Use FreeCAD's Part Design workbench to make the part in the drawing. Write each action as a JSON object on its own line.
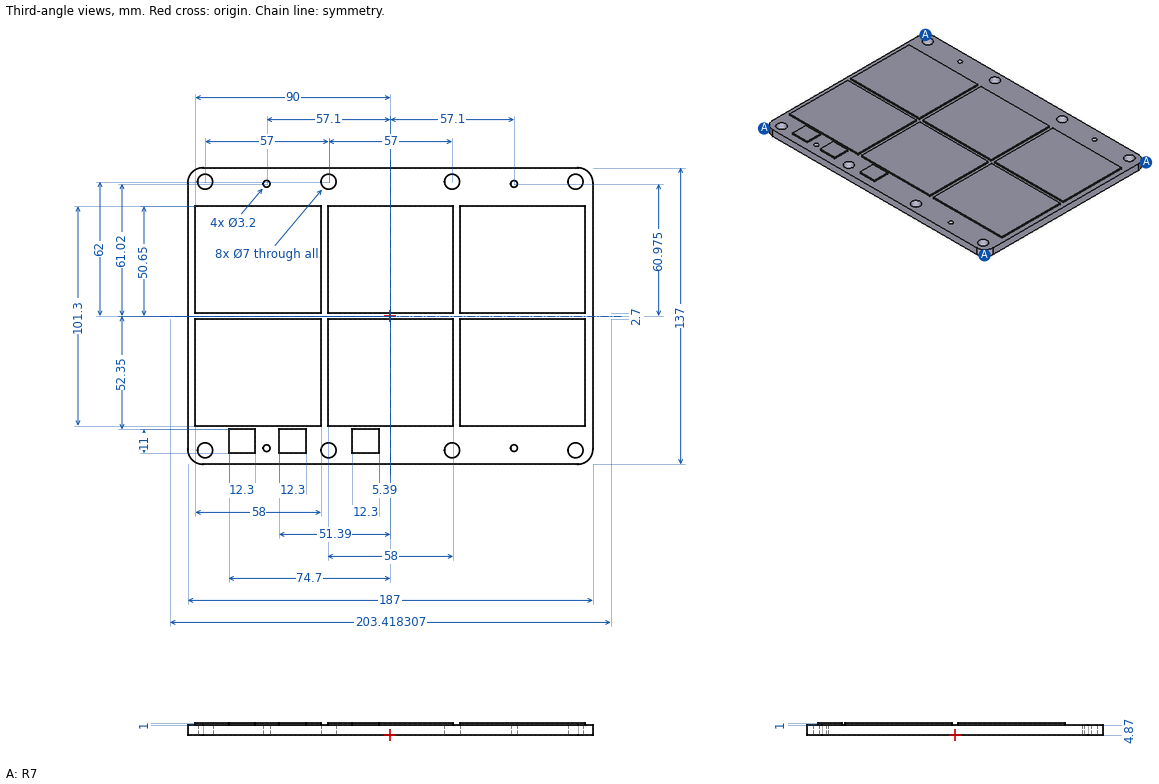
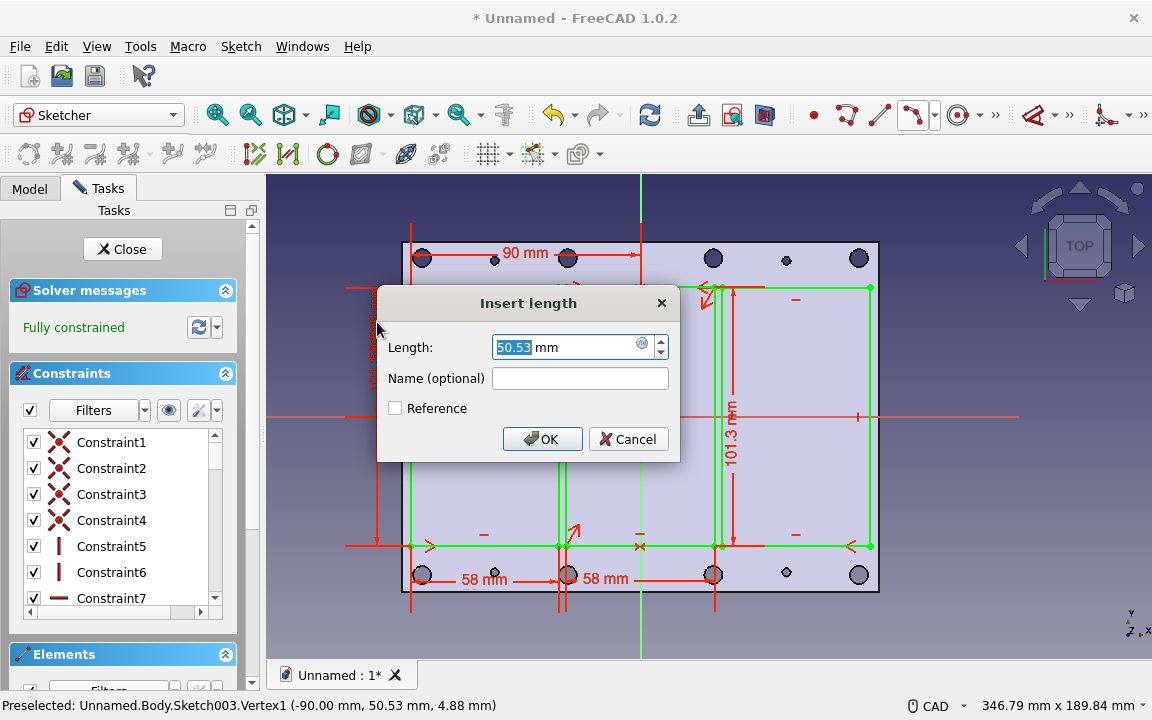
{"action": "type", "text": "50.65"}
{"action": "key", "text": "Return"}
{"action": "key", "text": "Escape"}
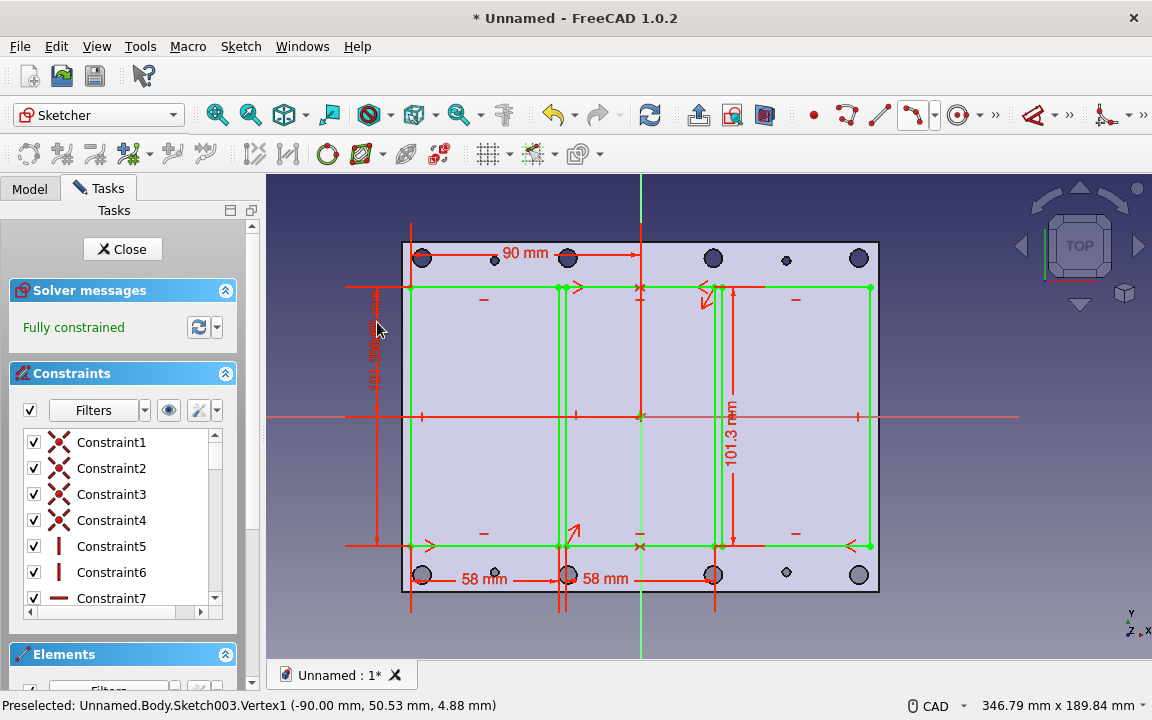
{"action": "left_click", "coordinate": [123, 249]}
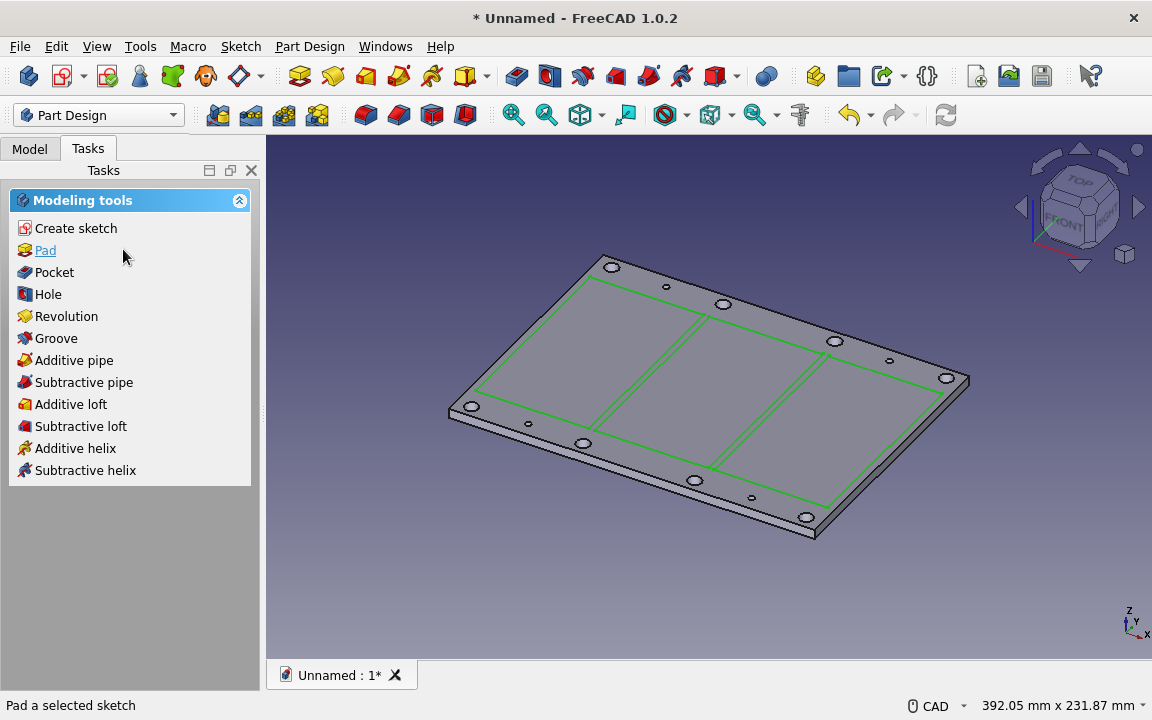
{"action": "left_click", "coordinate": [300, 76]}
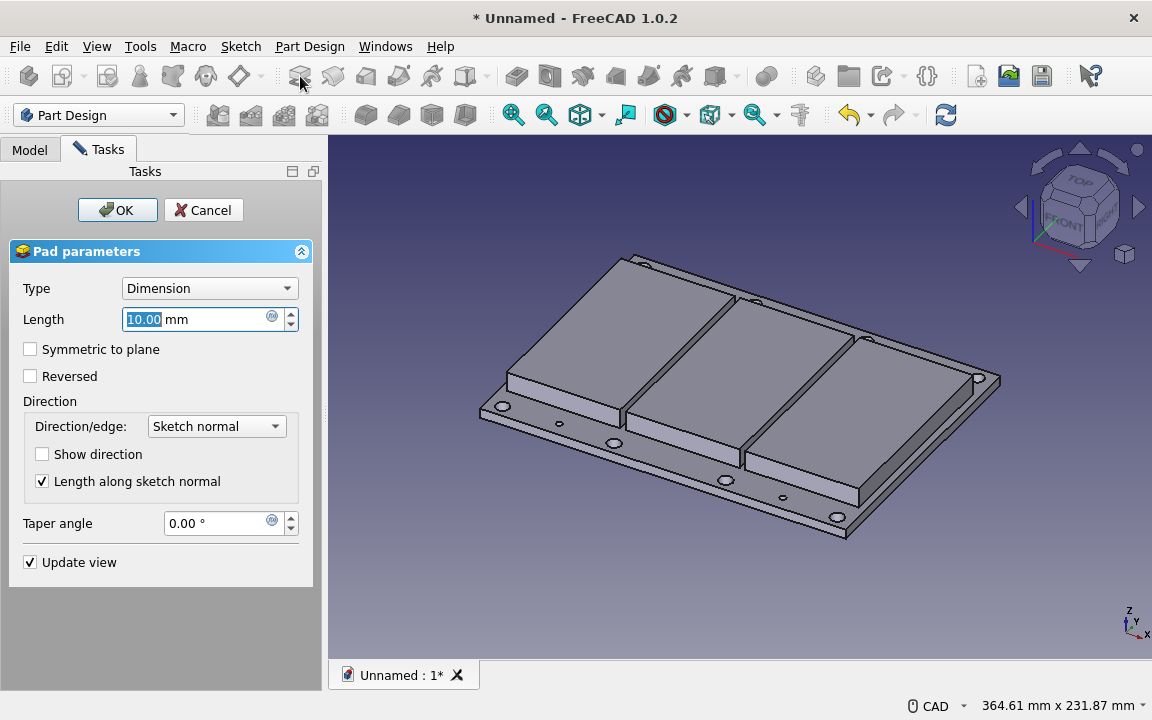
{"action": "type", "text": "1"}
{"action": "key", "text": "Tab"}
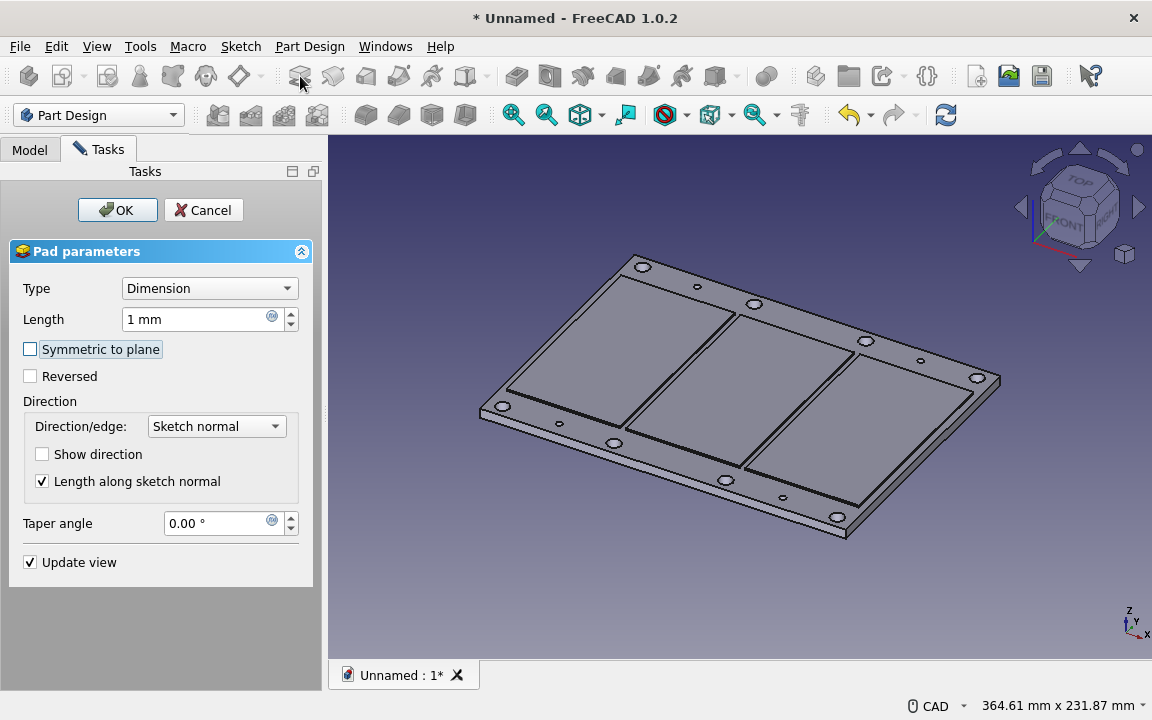
{"action": "left_click", "coordinate": [118, 210]}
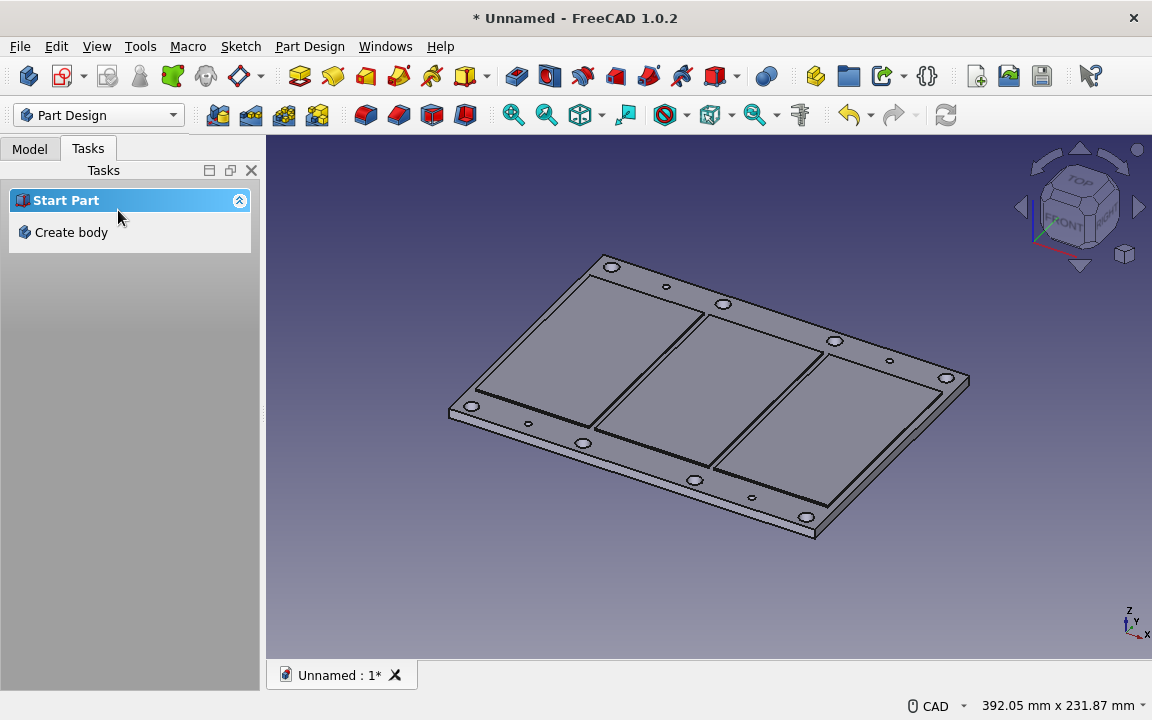
{"action": "left_click", "coordinate": [643, 457]}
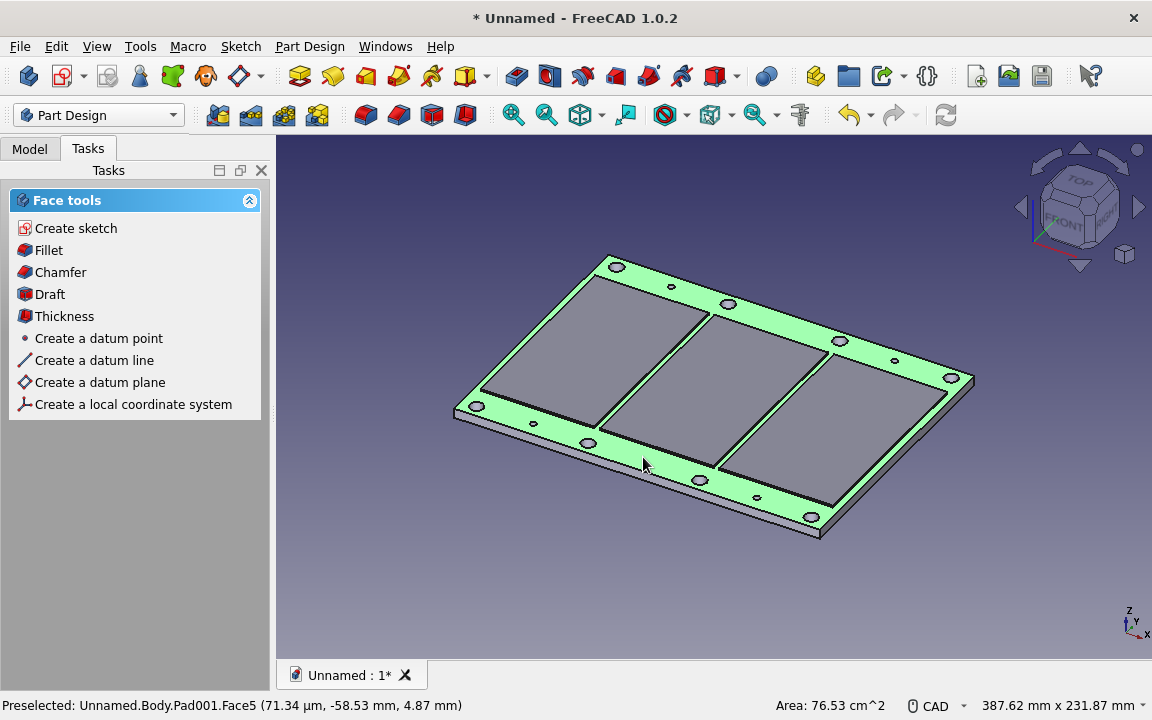
{"action": "left_click", "coordinate": [62, 76]}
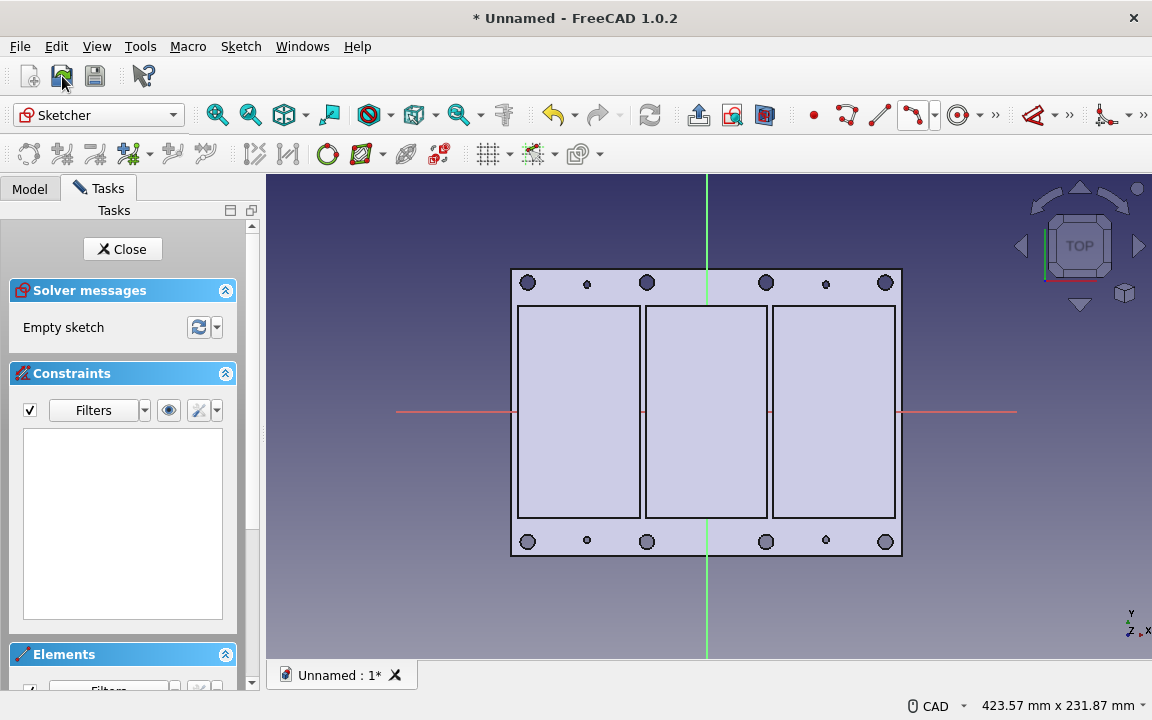
{"action": "key", "text": "q s"}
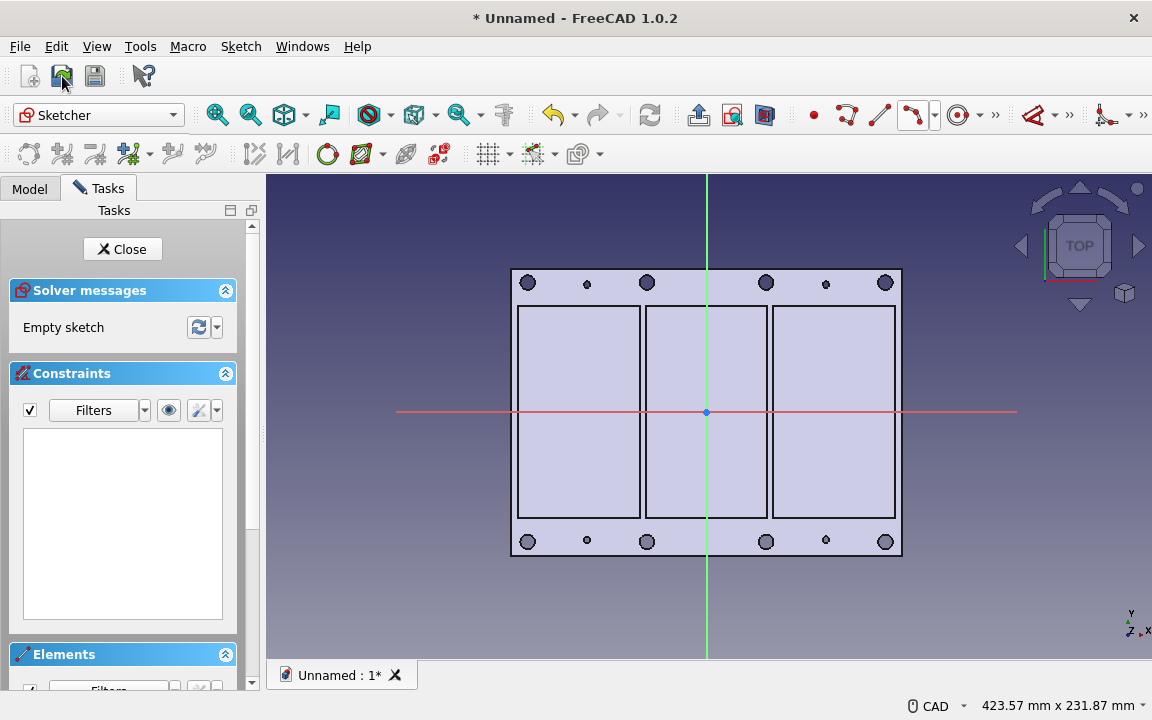
{"action": "scroll", "coordinate": [619, 529], "scroll_direction": "up", "scroll_amount": 4}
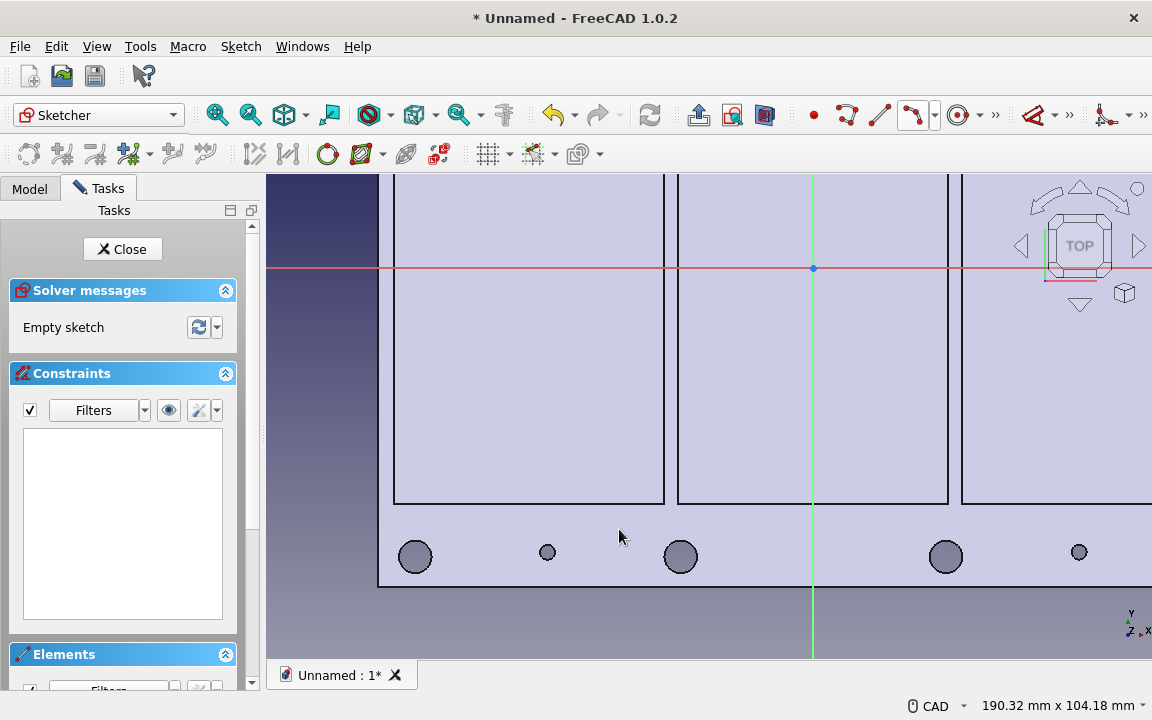
{"action": "key", "text": "g r"}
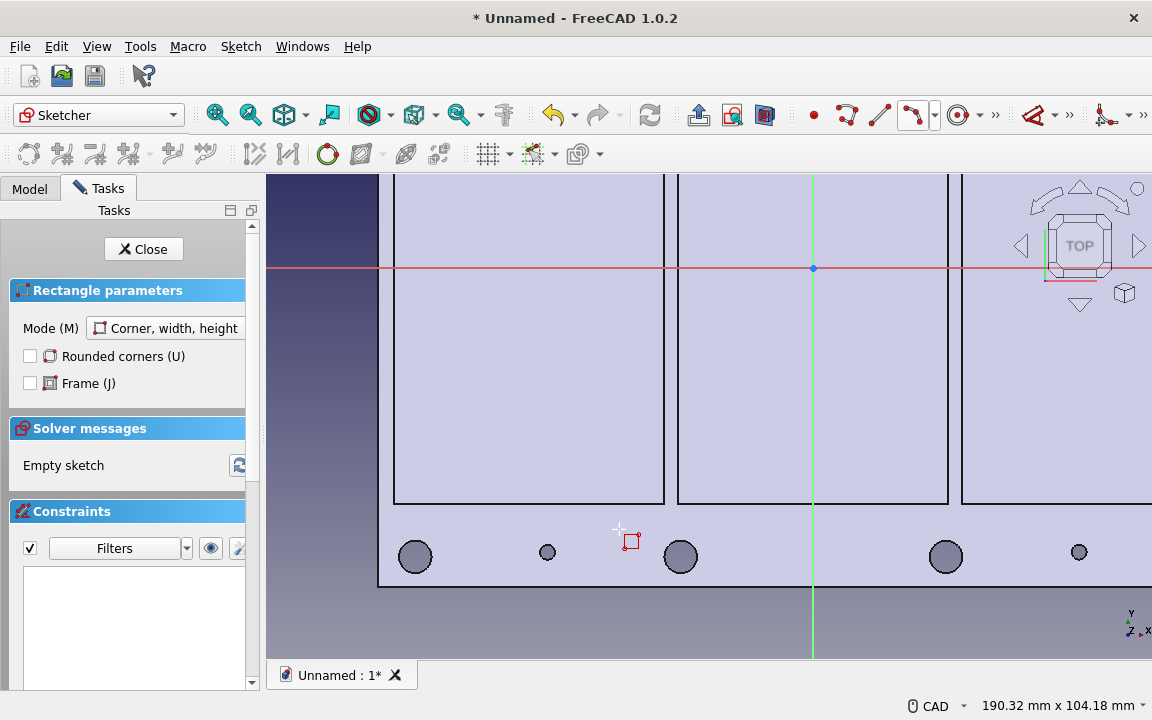
{"action": "left_click", "coordinate": [466, 512]}
{"action": "left_click", "coordinate": [523, 563]}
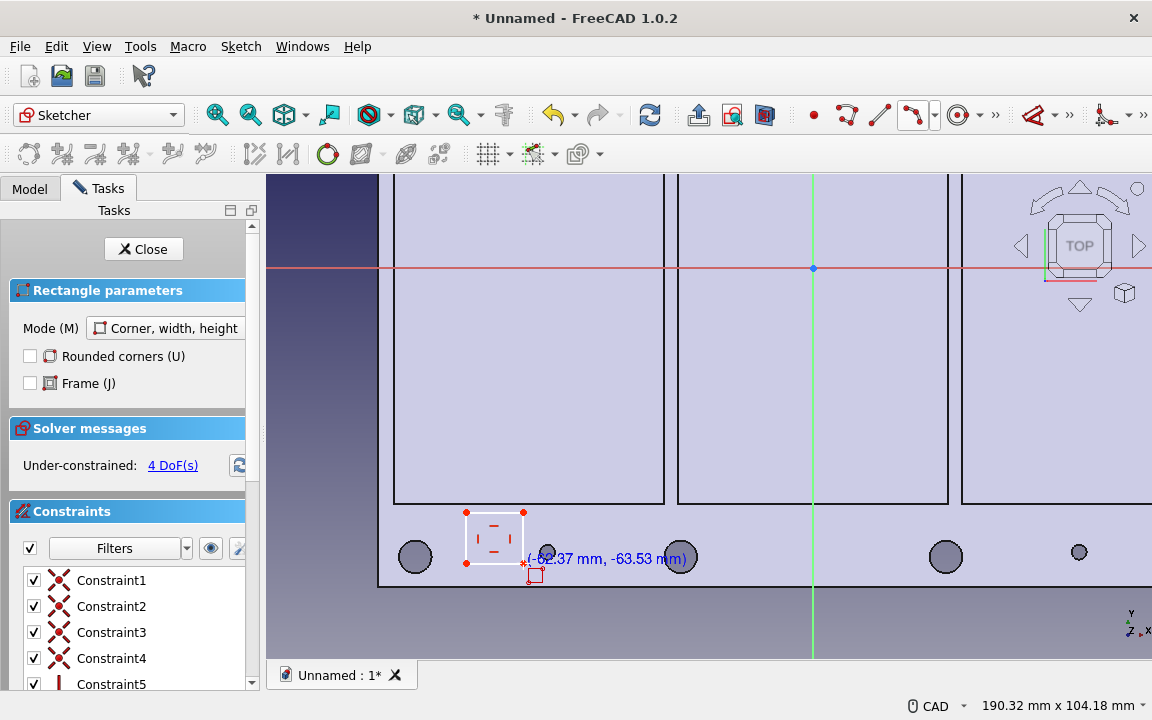
{"action": "left_click", "coordinate": [574, 512]}
{"action": "left_click", "coordinate": [631, 563]}